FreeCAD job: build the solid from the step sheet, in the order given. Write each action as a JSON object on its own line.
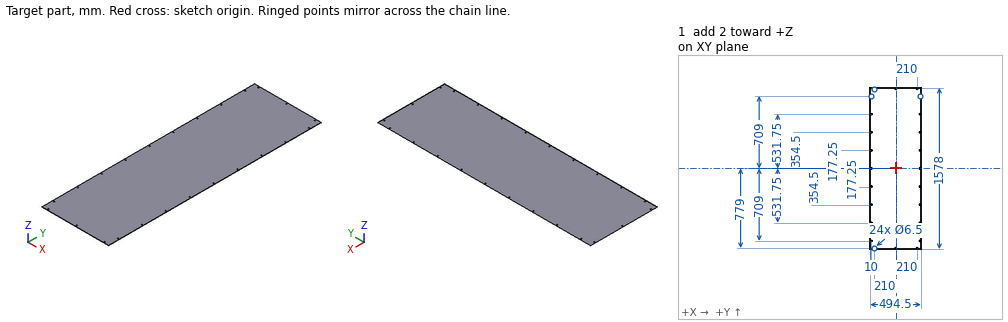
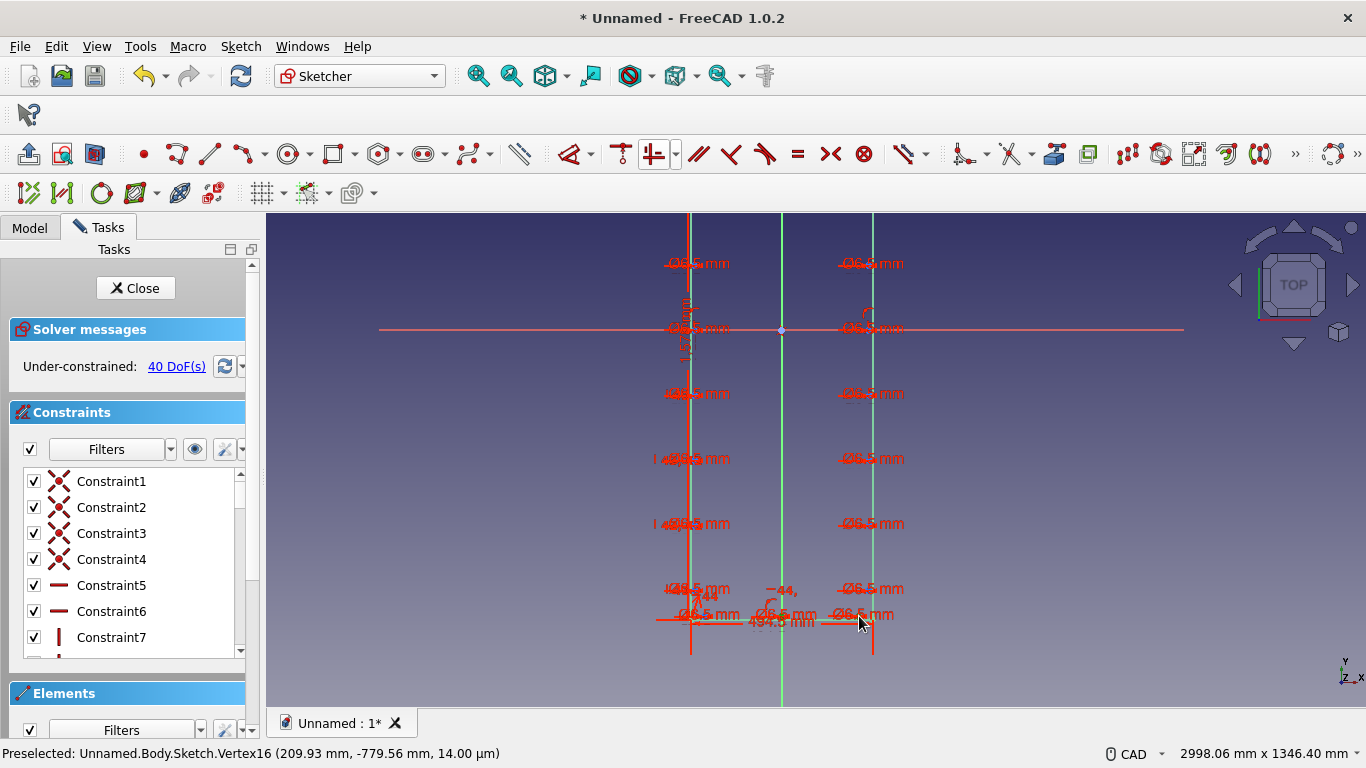
{"action": "left_click", "coordinate": [676, 154]}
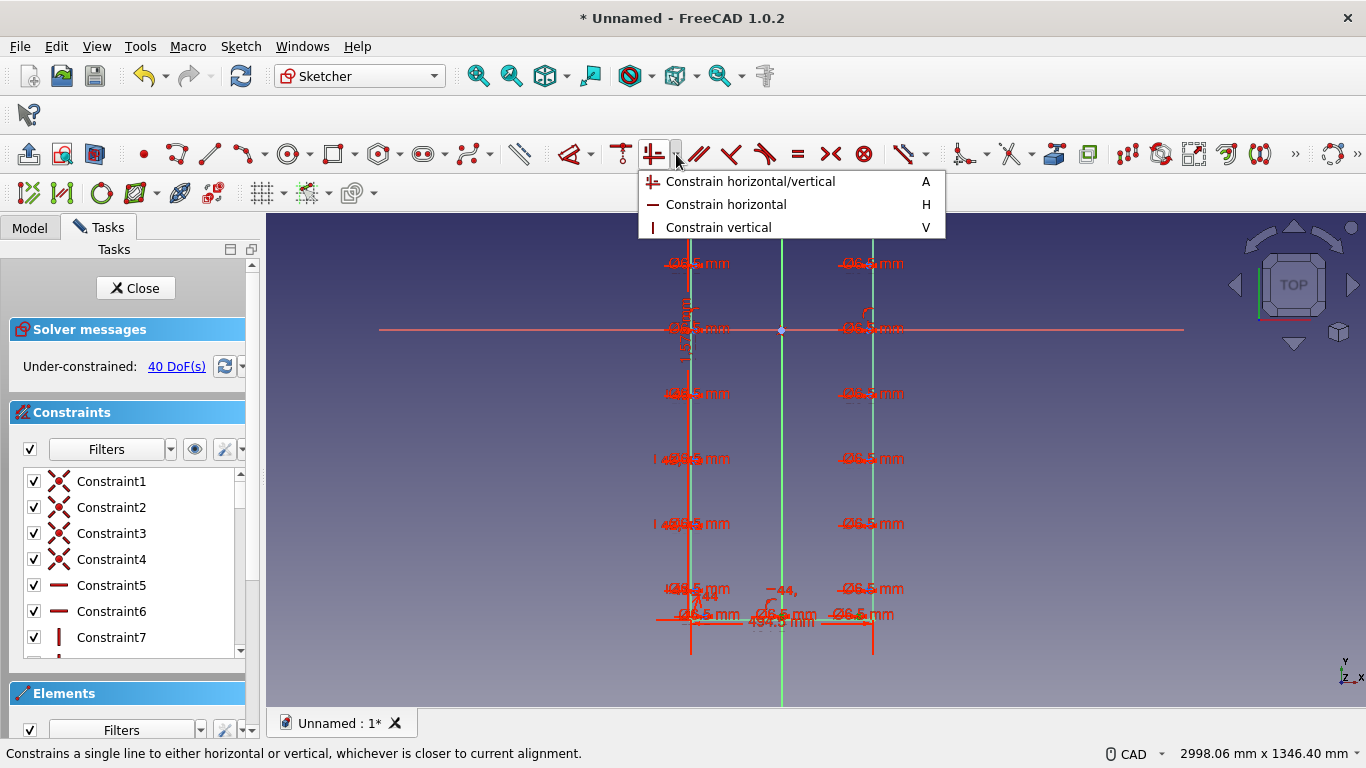
{"action": "left_click", "coordinate": [792, 204]}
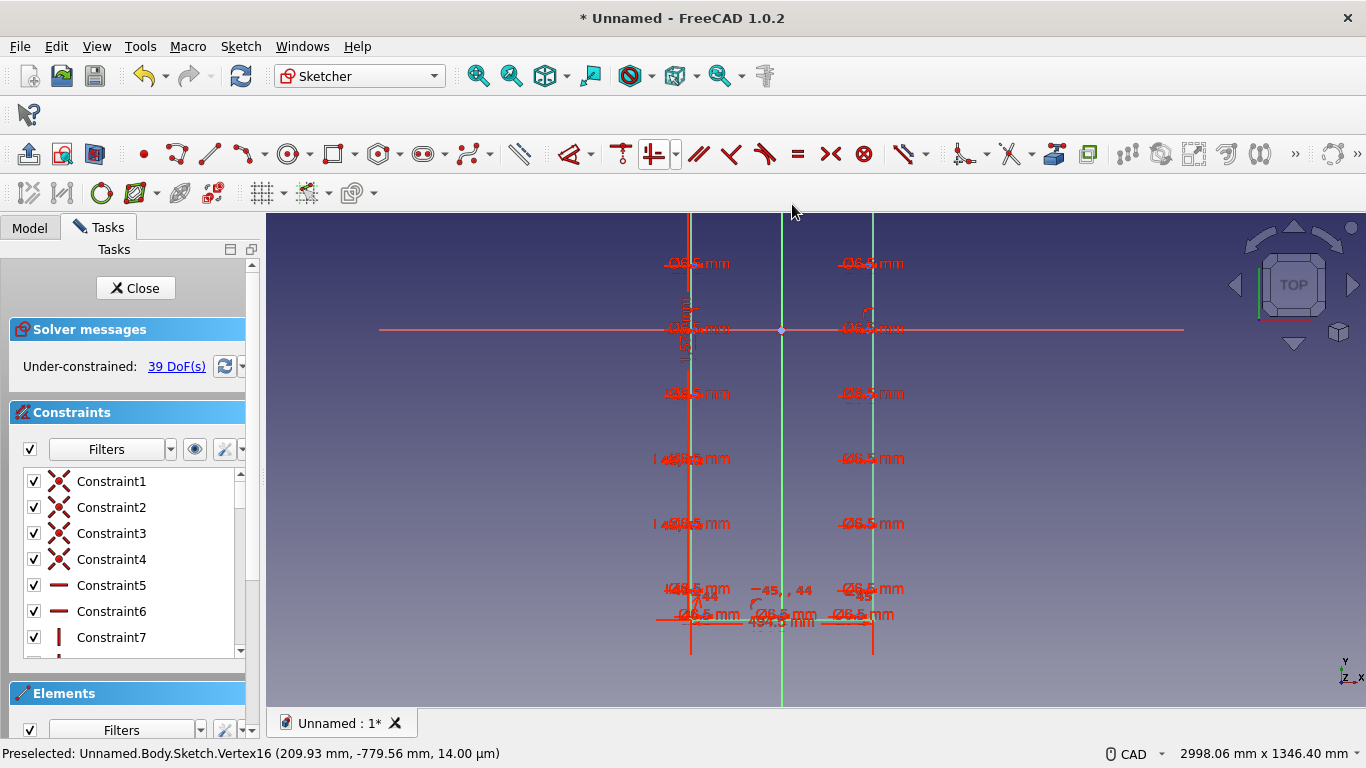
{"action": "left_click", "coordinate": [695, 591]}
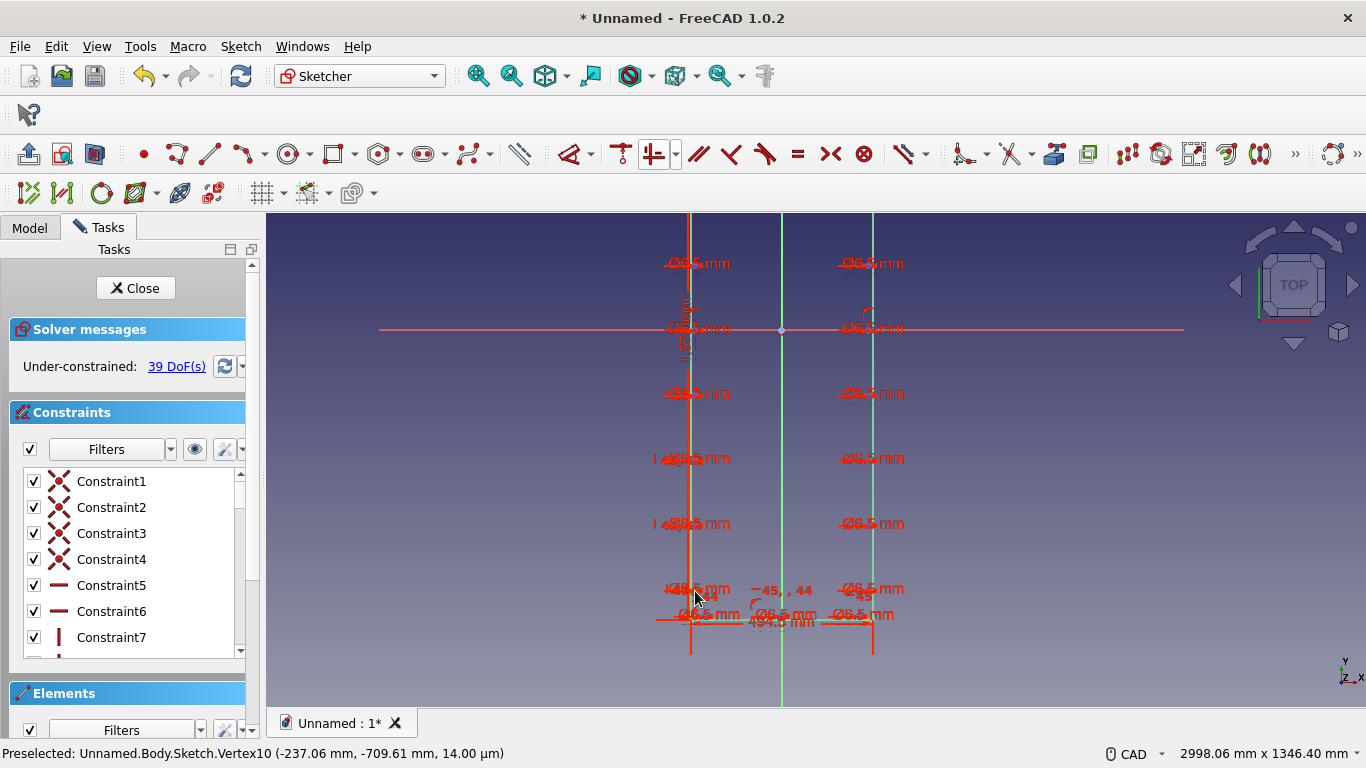
{"action": "scroll", "coordinate": [869, 591], "scroll_direction": "up", "scroll_amount": 4}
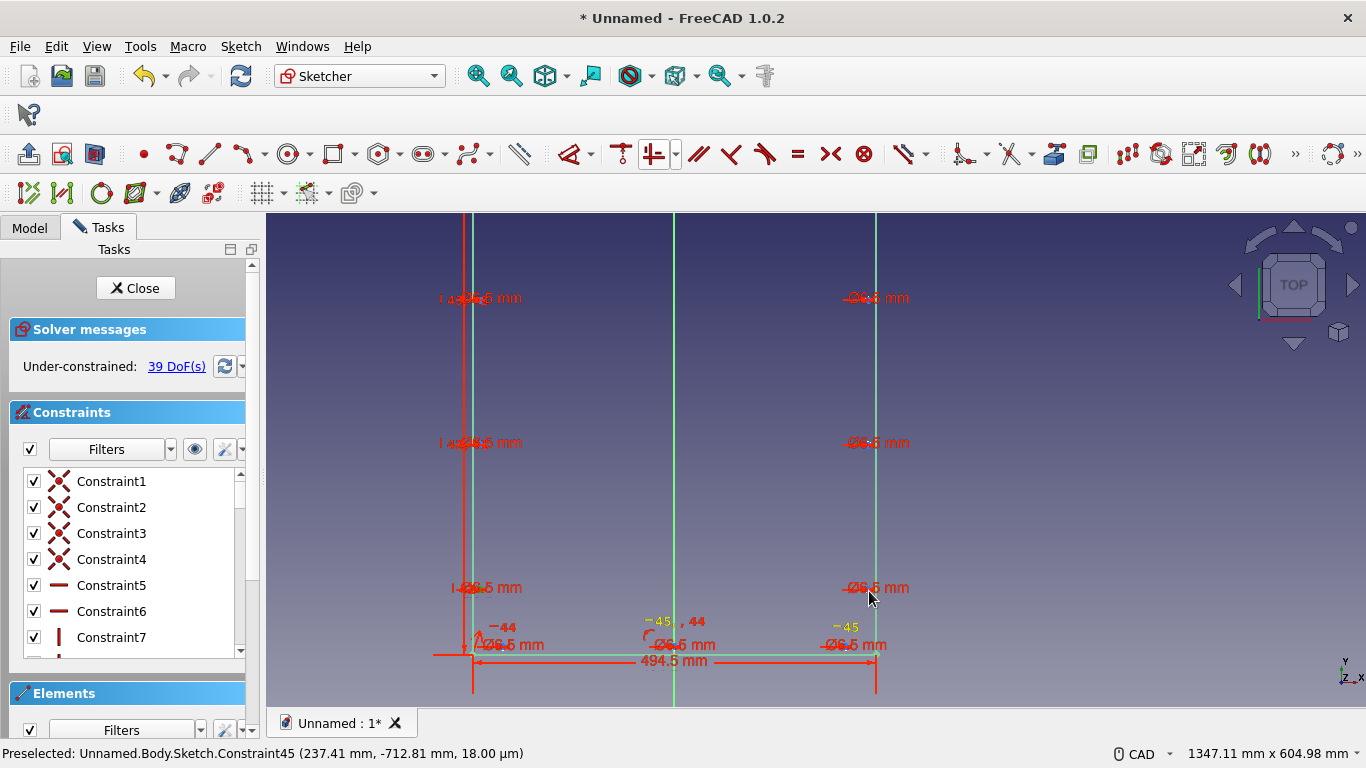
{"action": "left_click", "coordinate": [868, 590]}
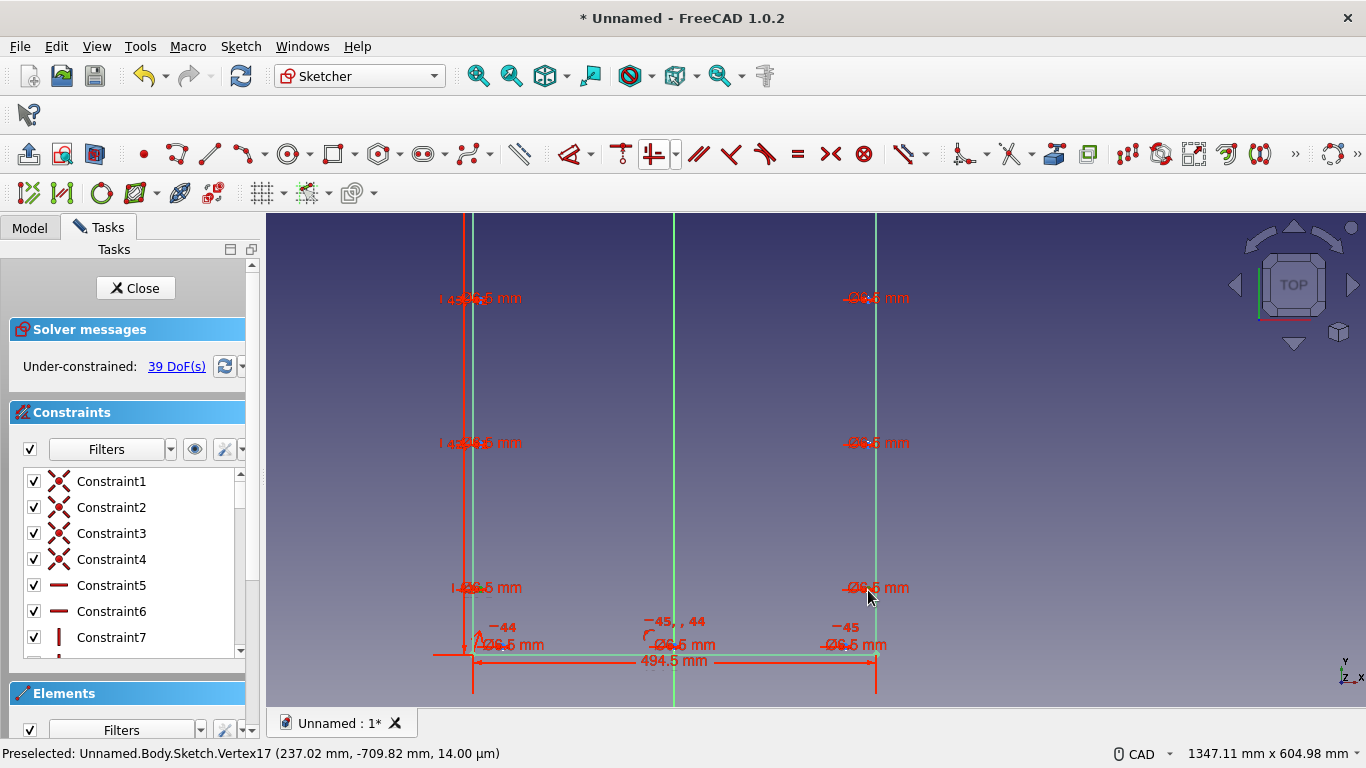
{"action": "key", "text": "h"}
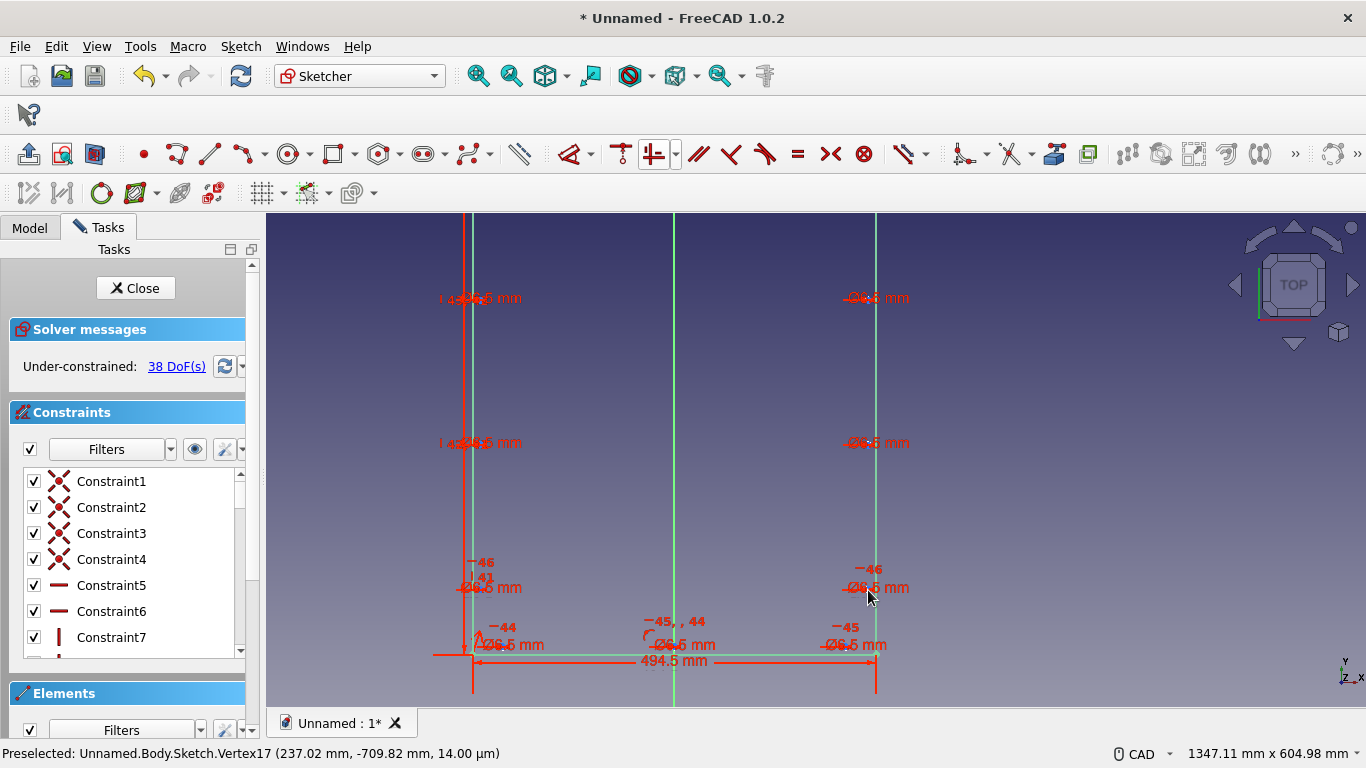
{"action": "scroll", "coordinate": [771, 607], "scroll_direction": "down", "scroll_amount": 7}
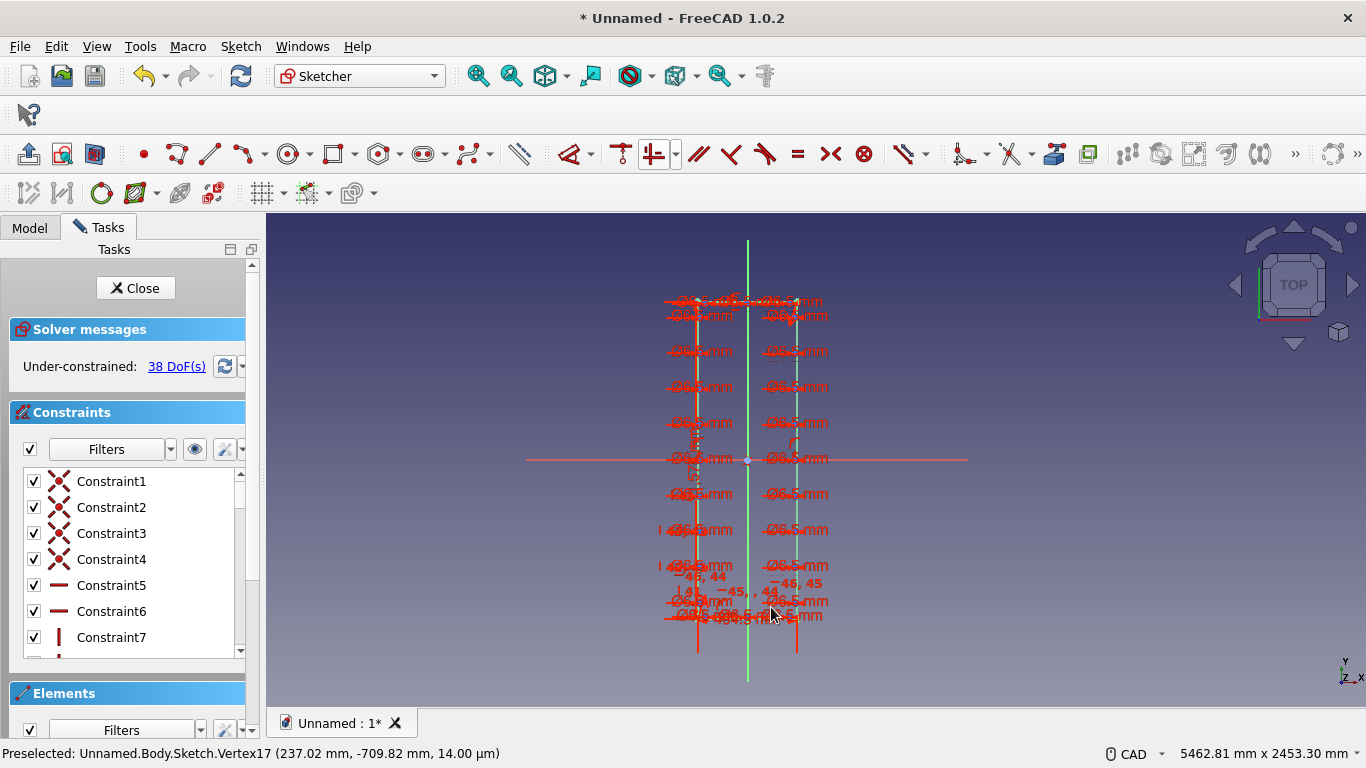
{"action": "left_click", "coordinate": [795, 603]}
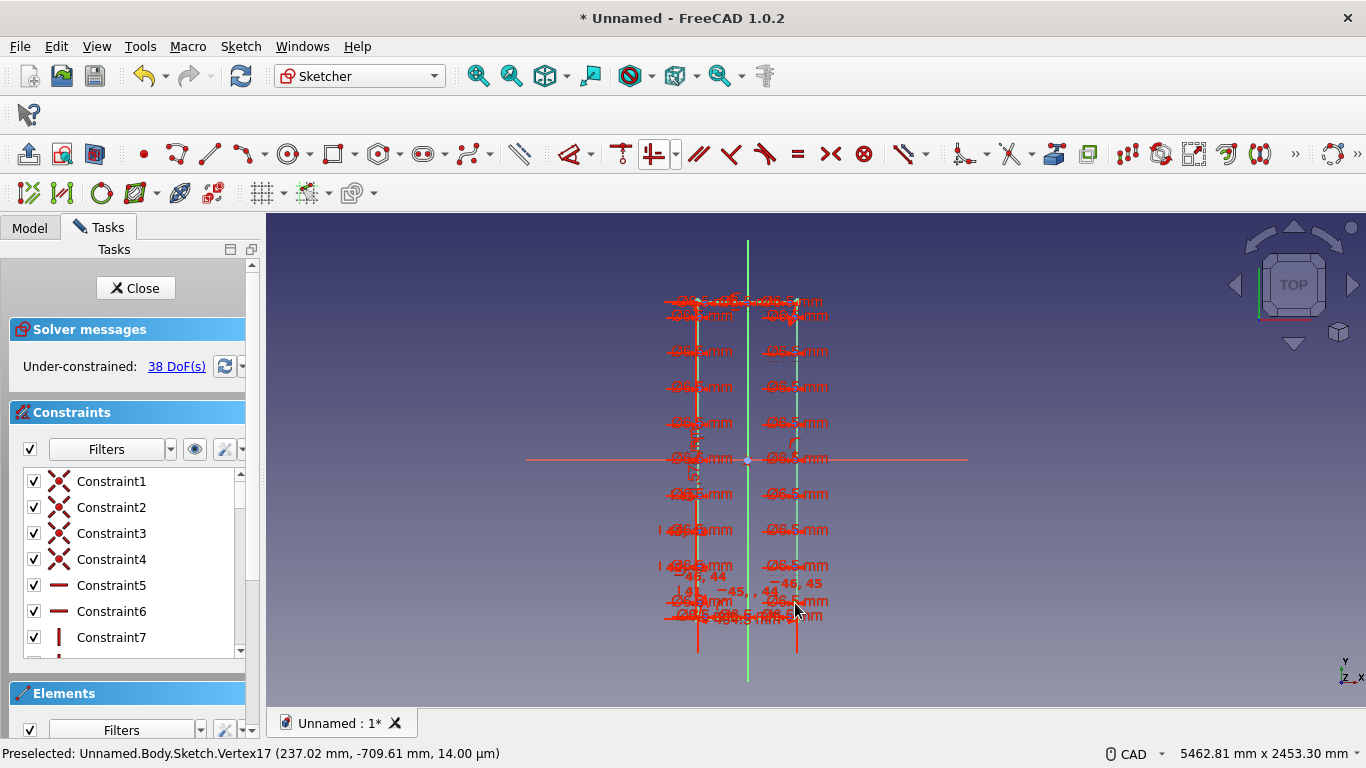
{"action": "left_click", "coordinate": [795, 568]}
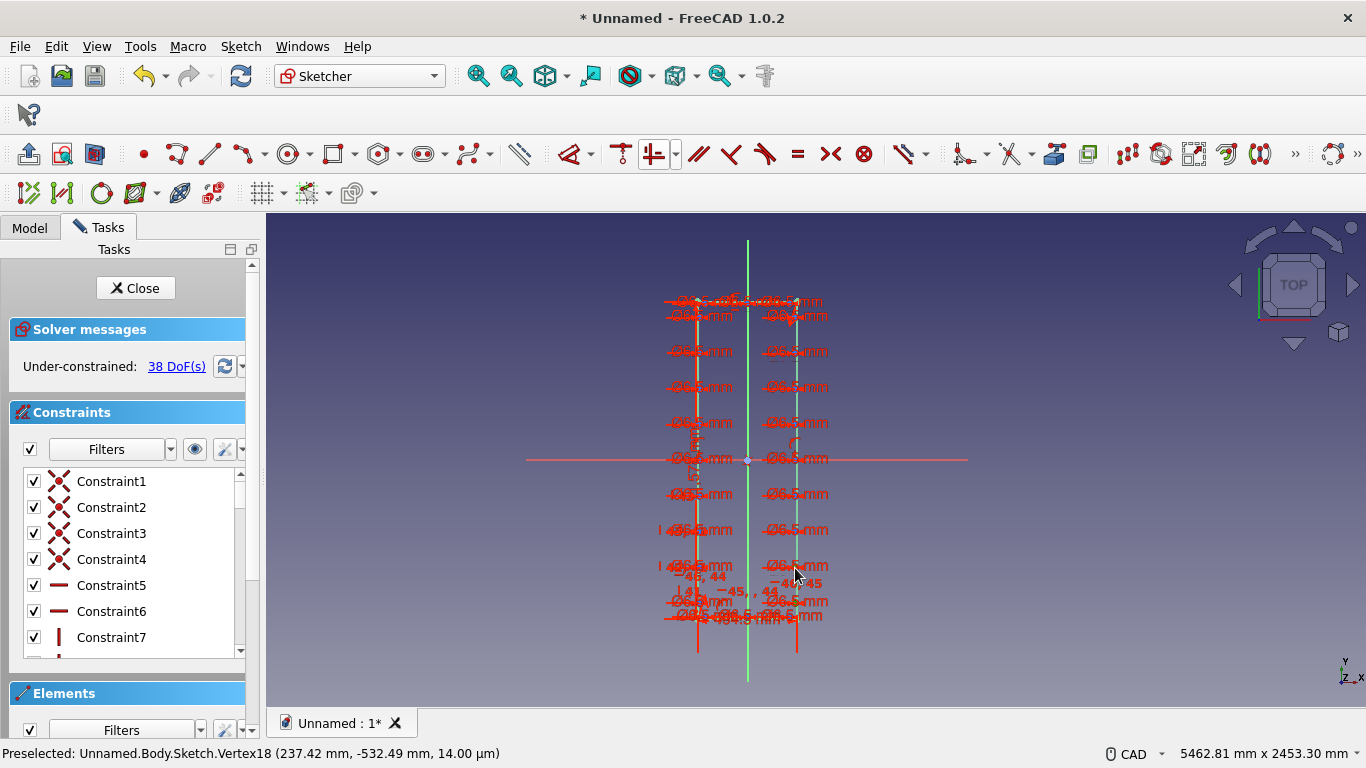
{"action": "left_click", "coordinate": [676, 154]}